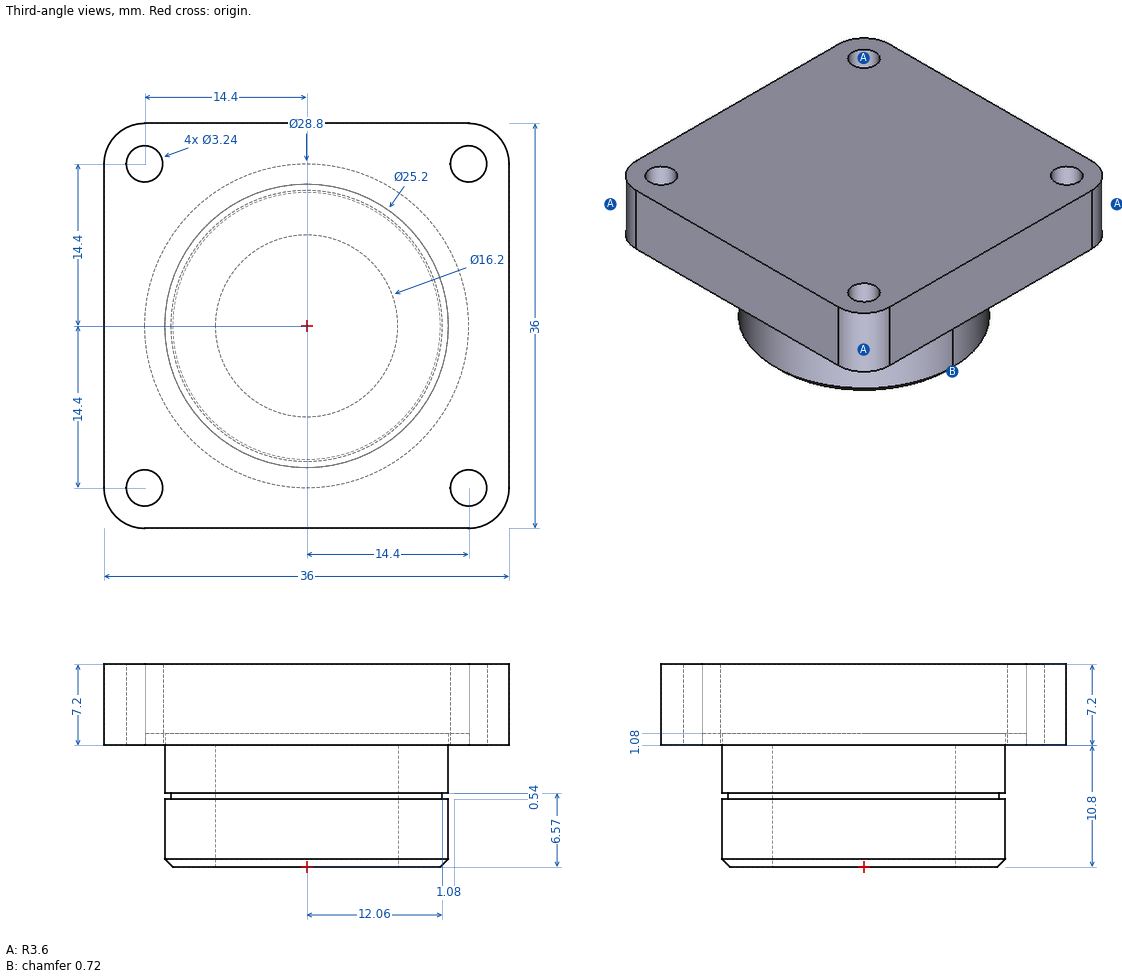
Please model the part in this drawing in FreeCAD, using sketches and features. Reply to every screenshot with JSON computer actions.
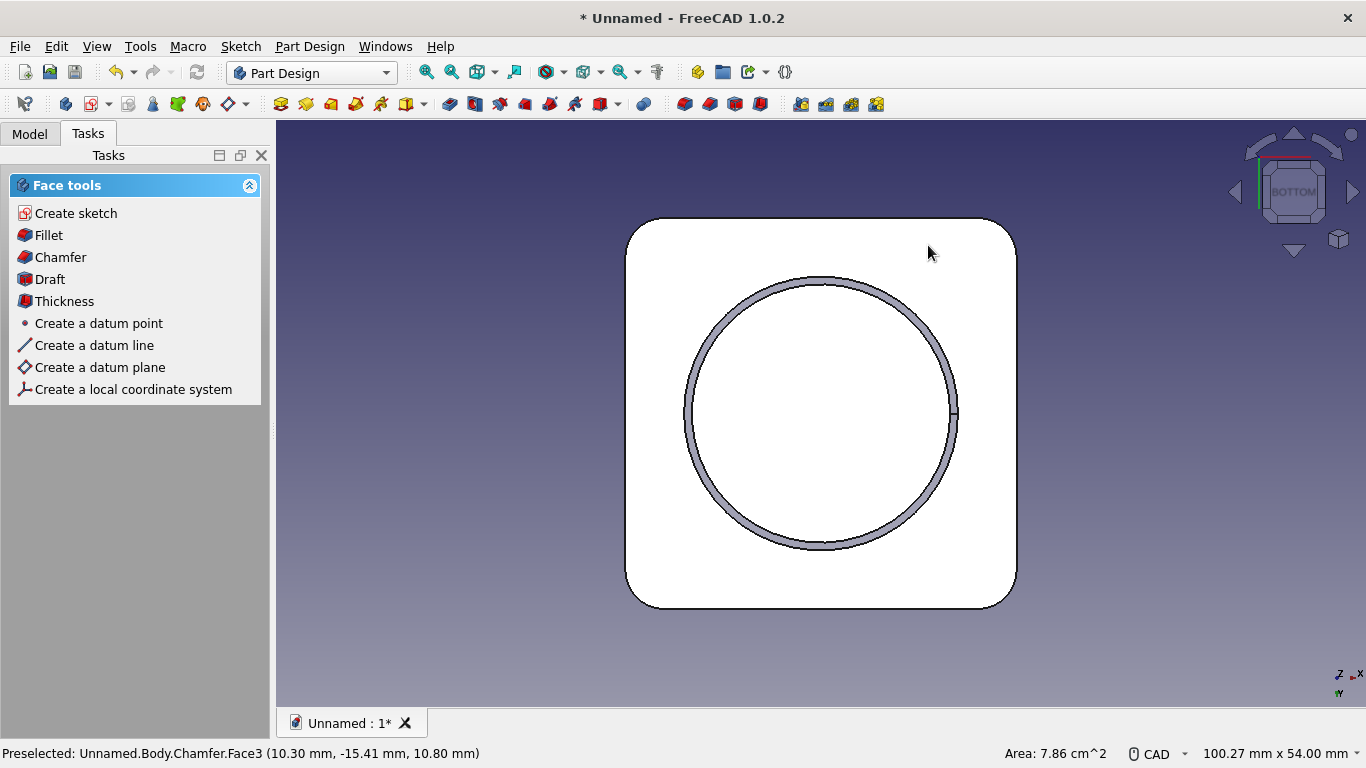
{"action": "left_click", "coordinate": [90, 104]}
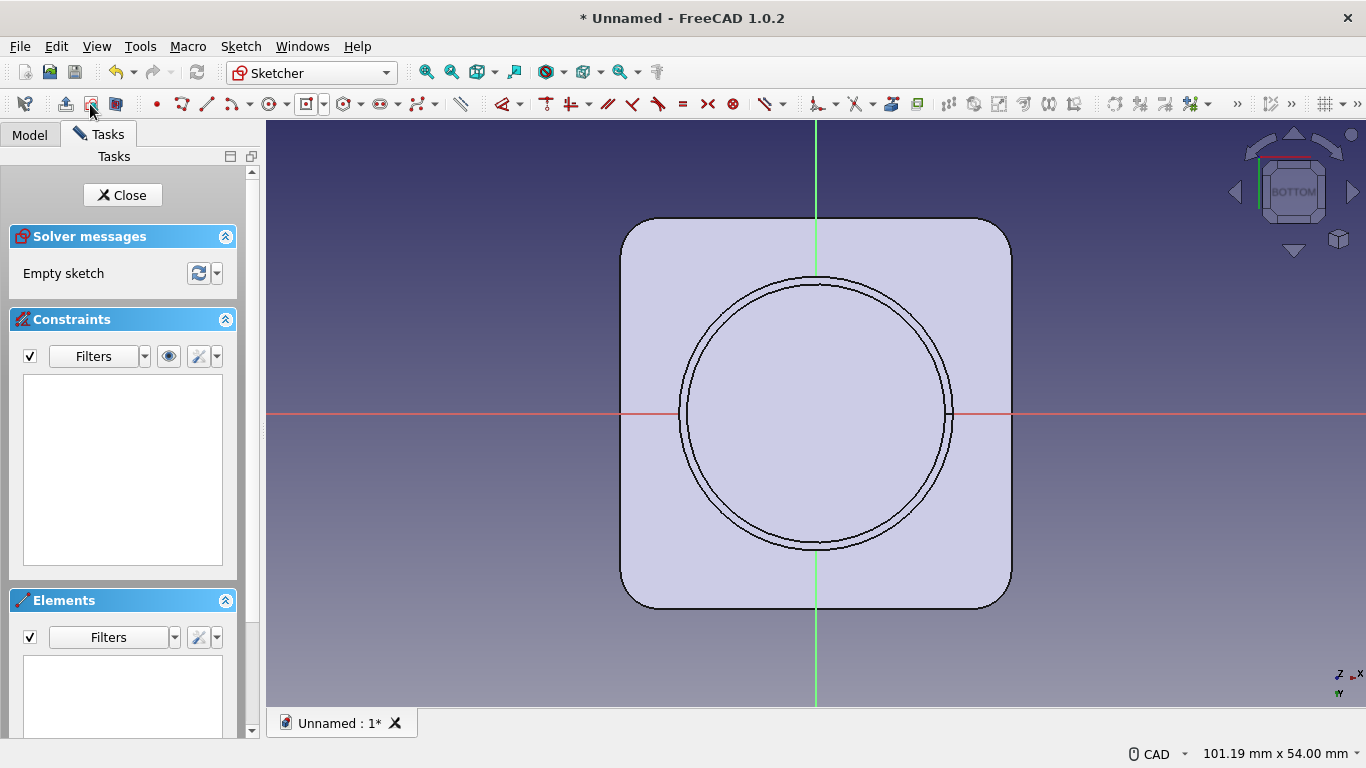
{"action": "left_click", "coordinate": [116, 104]}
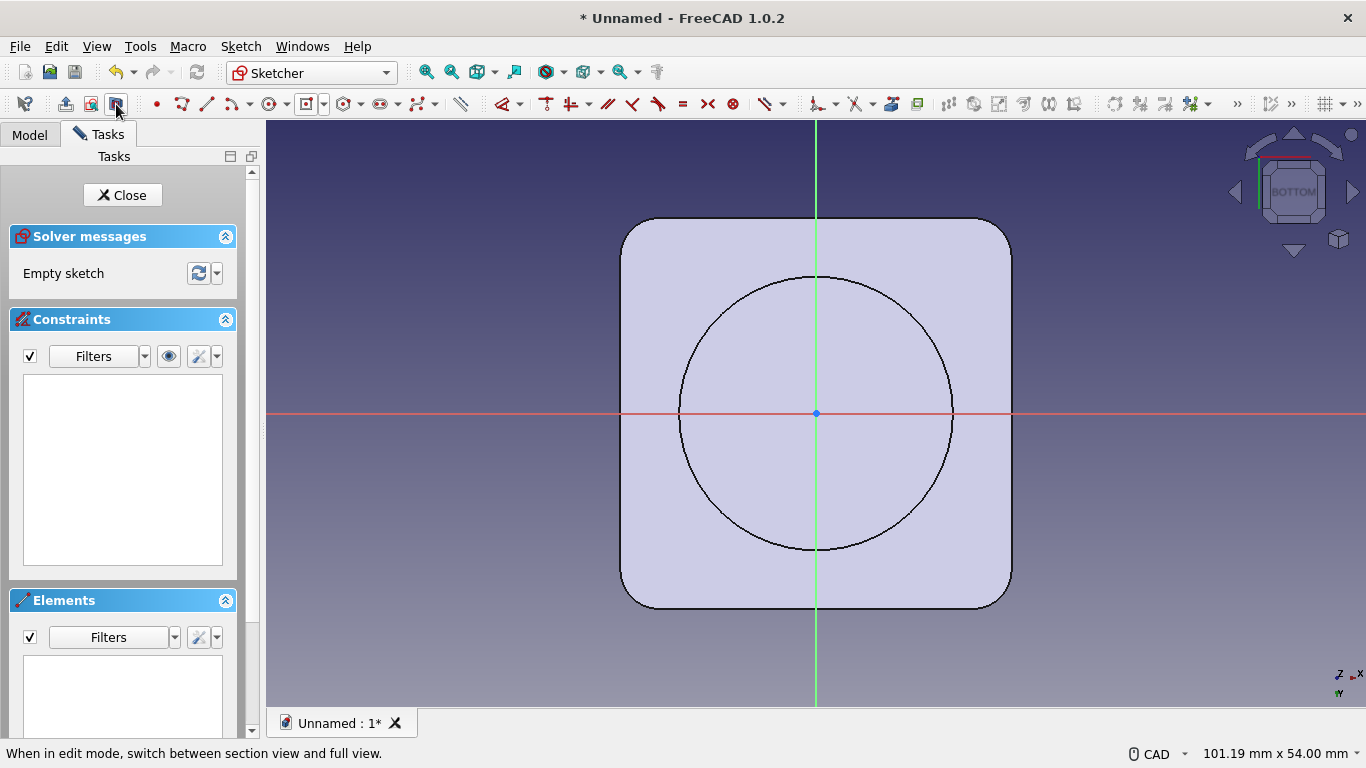
{"action": "key", "text": "g c"}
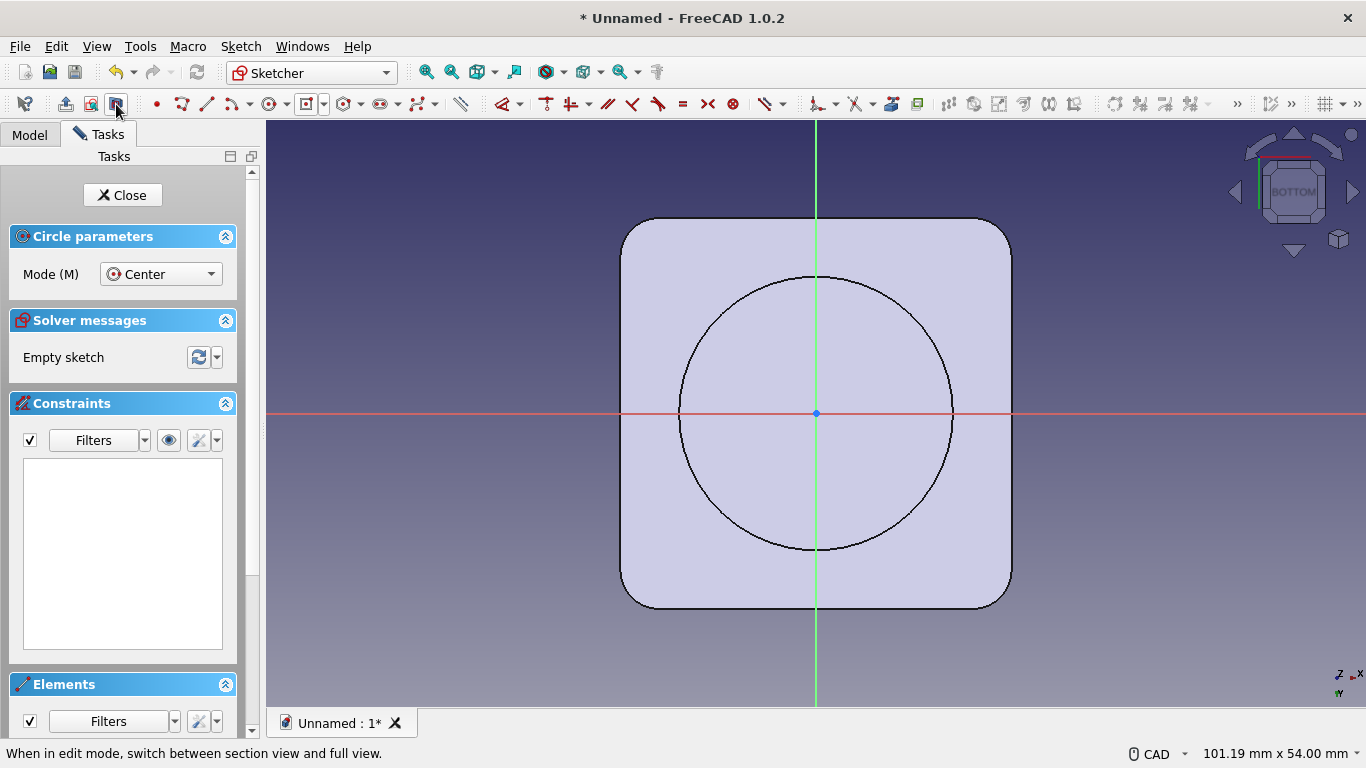
{"action": "left_click", "coordinate": [816, 414]}
{"action": "mouse_move", "coordinate": [927, 303]}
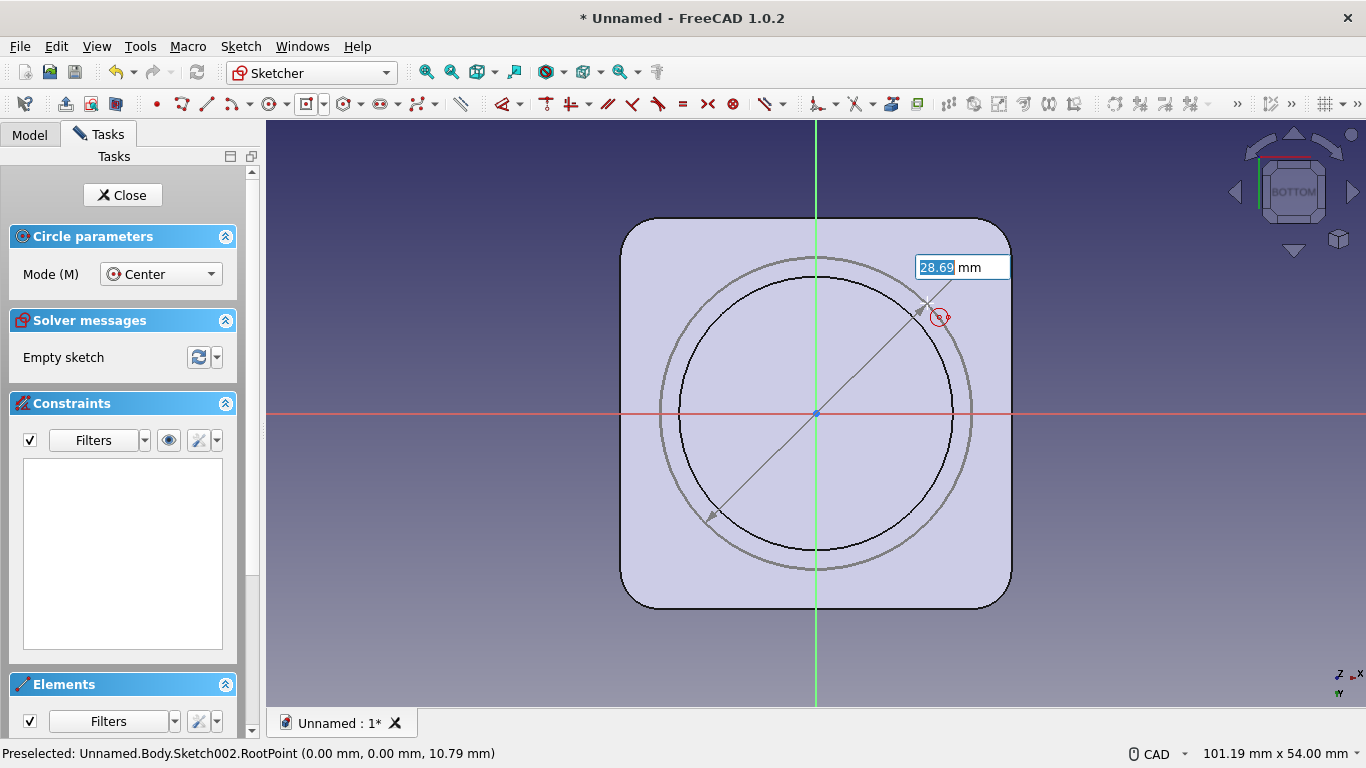
{"action": "type", "text": "28.8"}
{"action": "key", "text": "Return"}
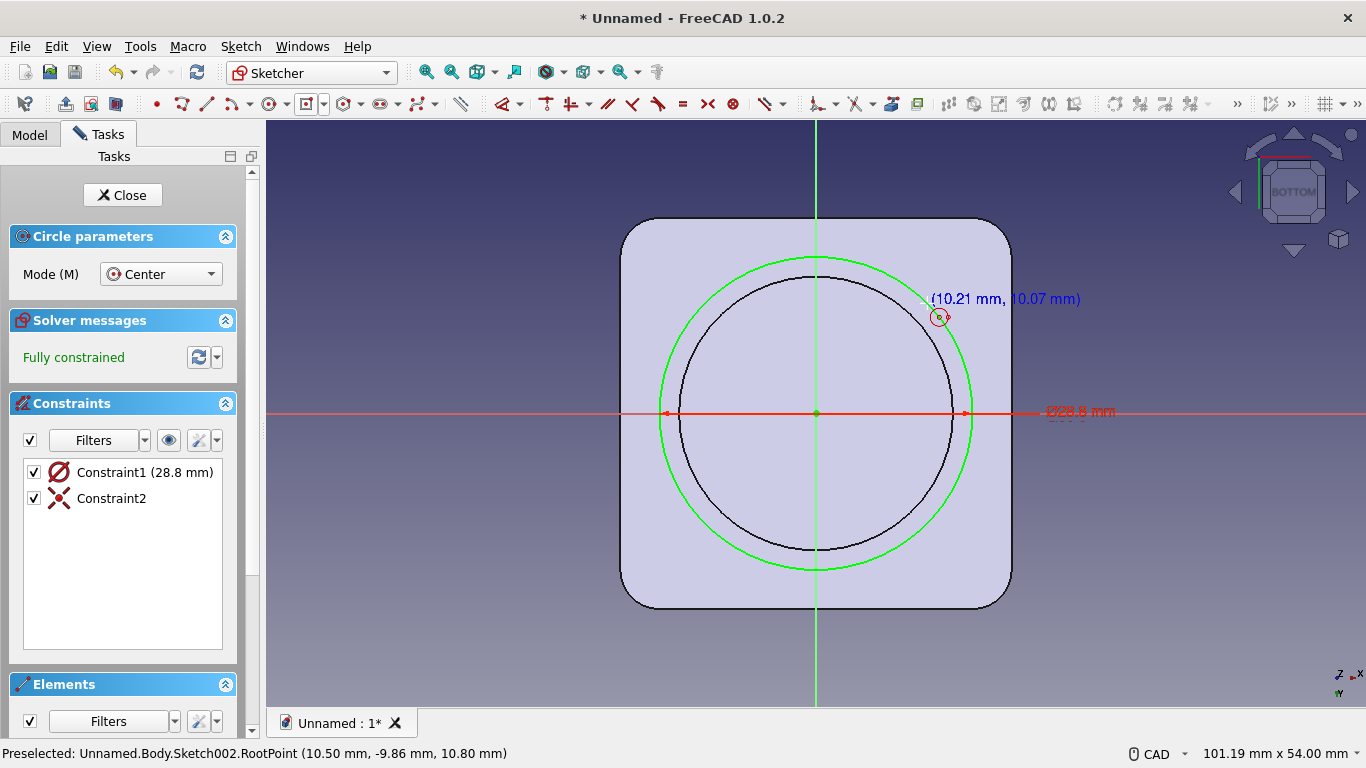
{"action": "left_click", "coordinate": [816, 414]}
{"action": "mouse_move", "coordinate": [913, 317]}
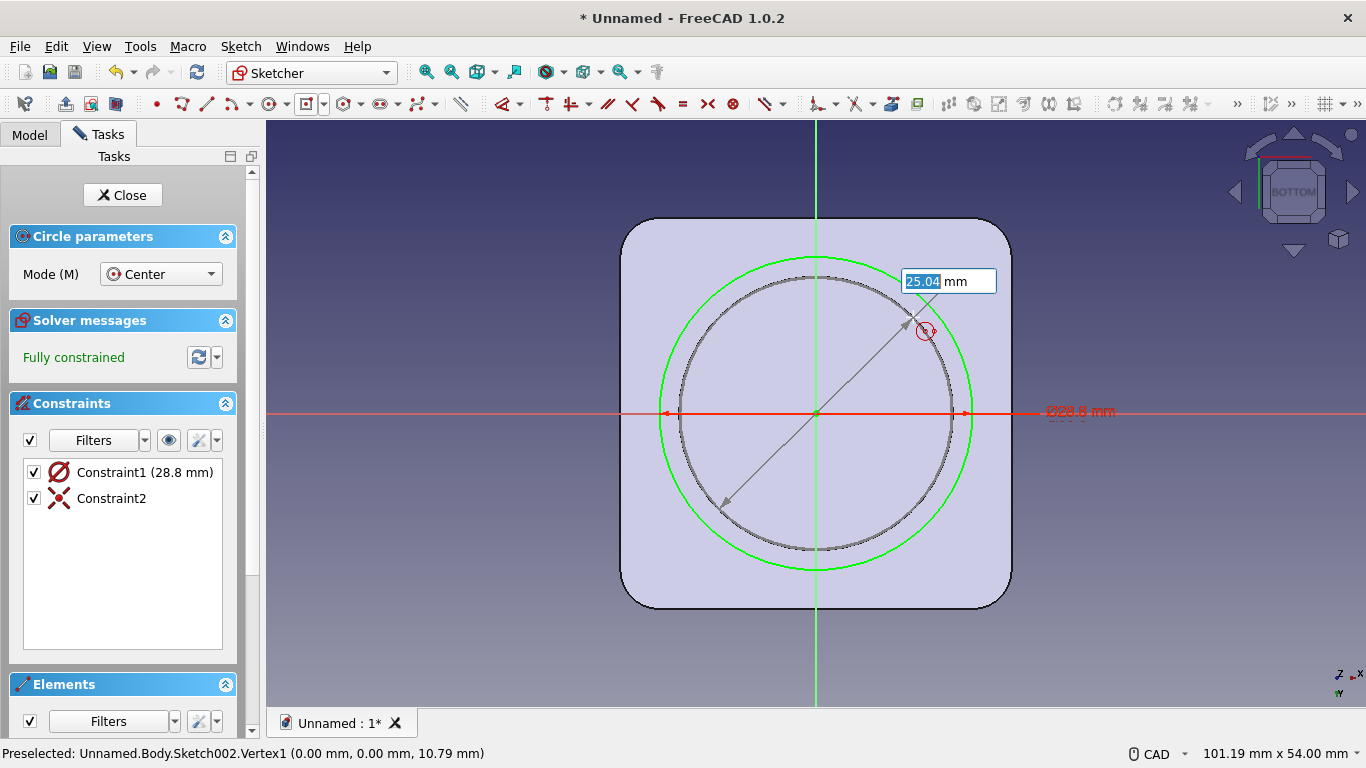
{"action": "type", "text": "25.2"}
{"action": "key", "text": "Return"}
{"action": "key", "text": "Escape"}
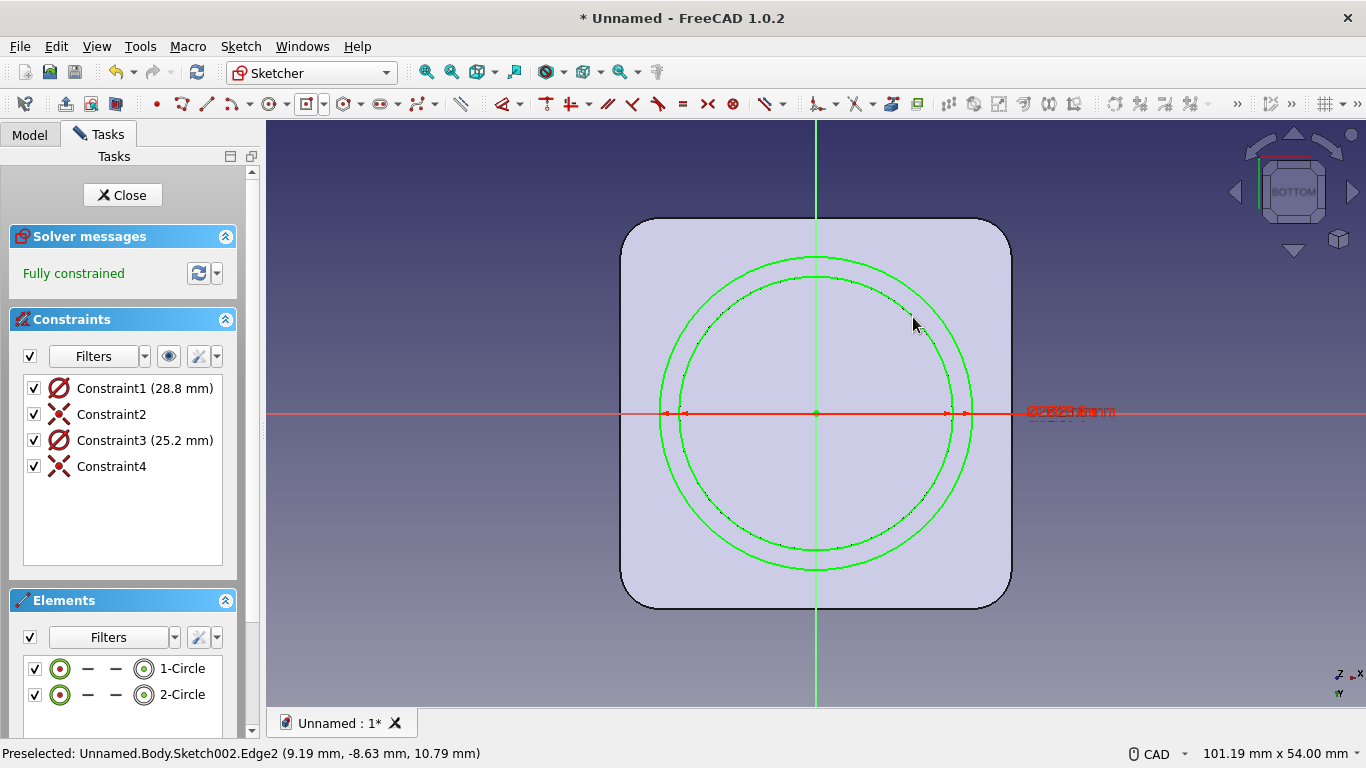
{"action": "left_click", "coordinate": [123, 195]}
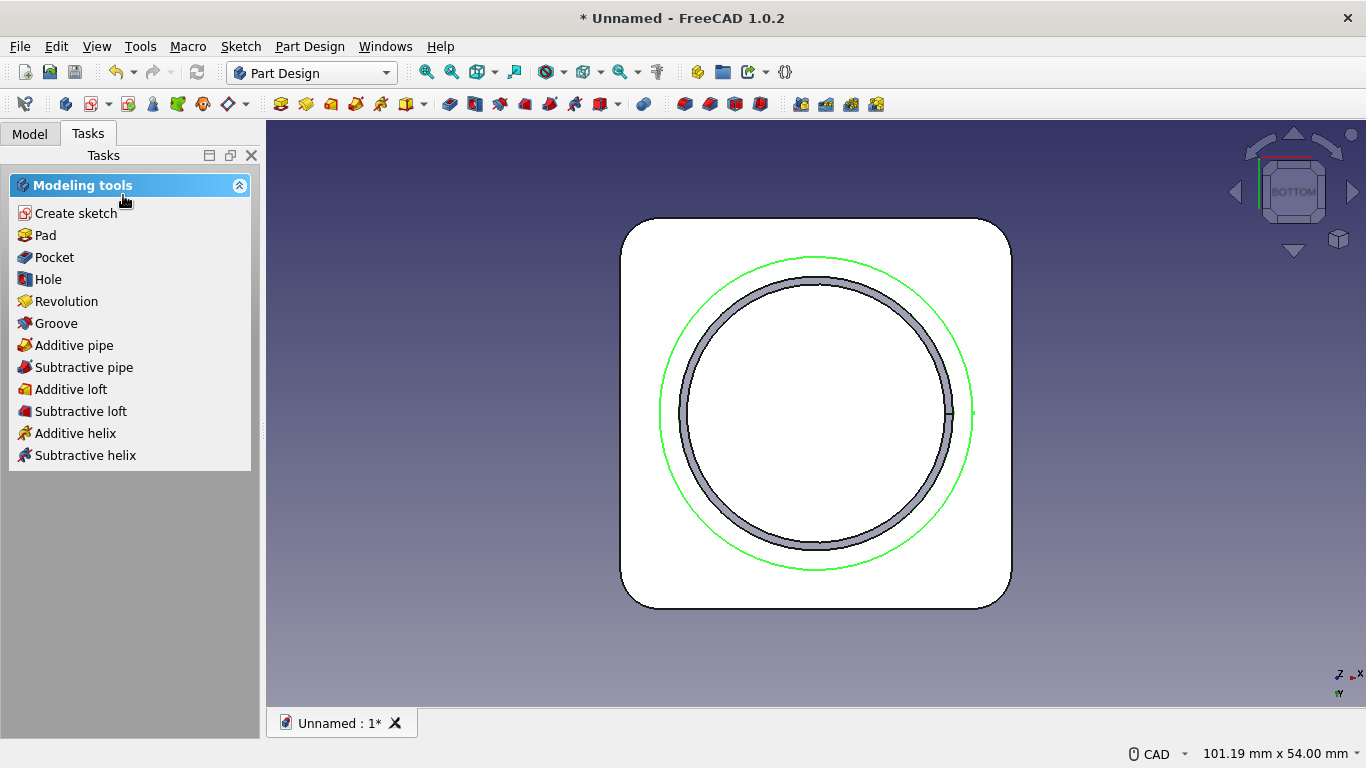
{"action": "left_click", "coordinate": [450, 104]}